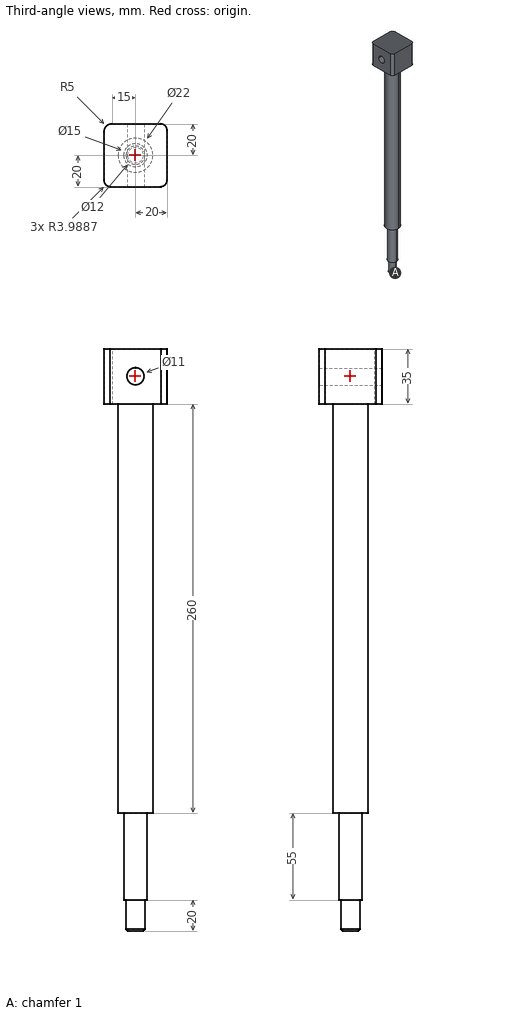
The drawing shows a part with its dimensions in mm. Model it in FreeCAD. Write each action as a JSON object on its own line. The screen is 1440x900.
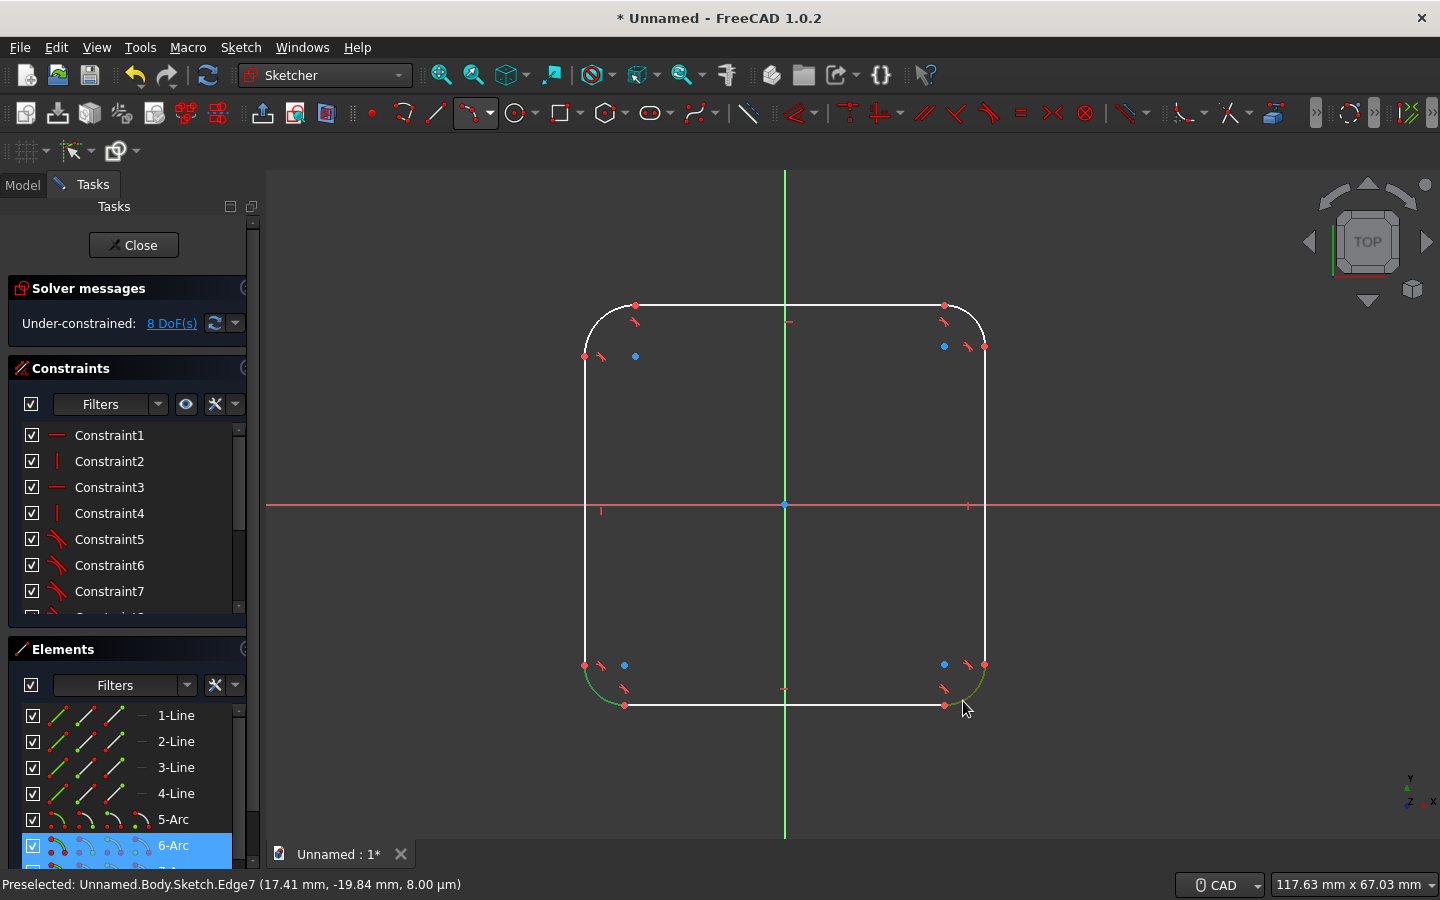
{"action": "left_click", "coordinate": [981, 328]}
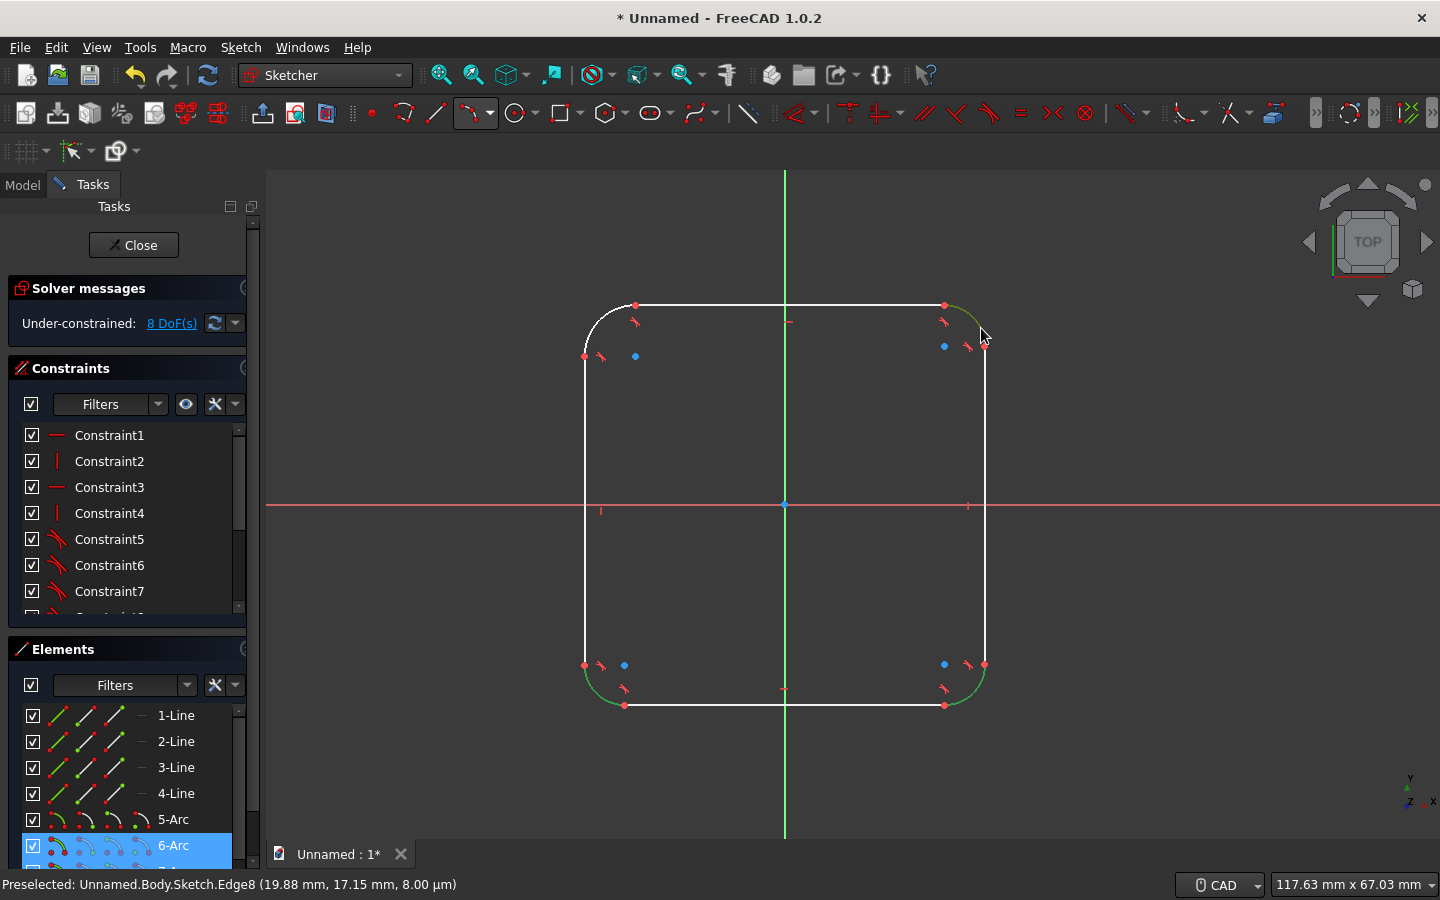
{"action": "left_click", "coordinate": [1022, 114]}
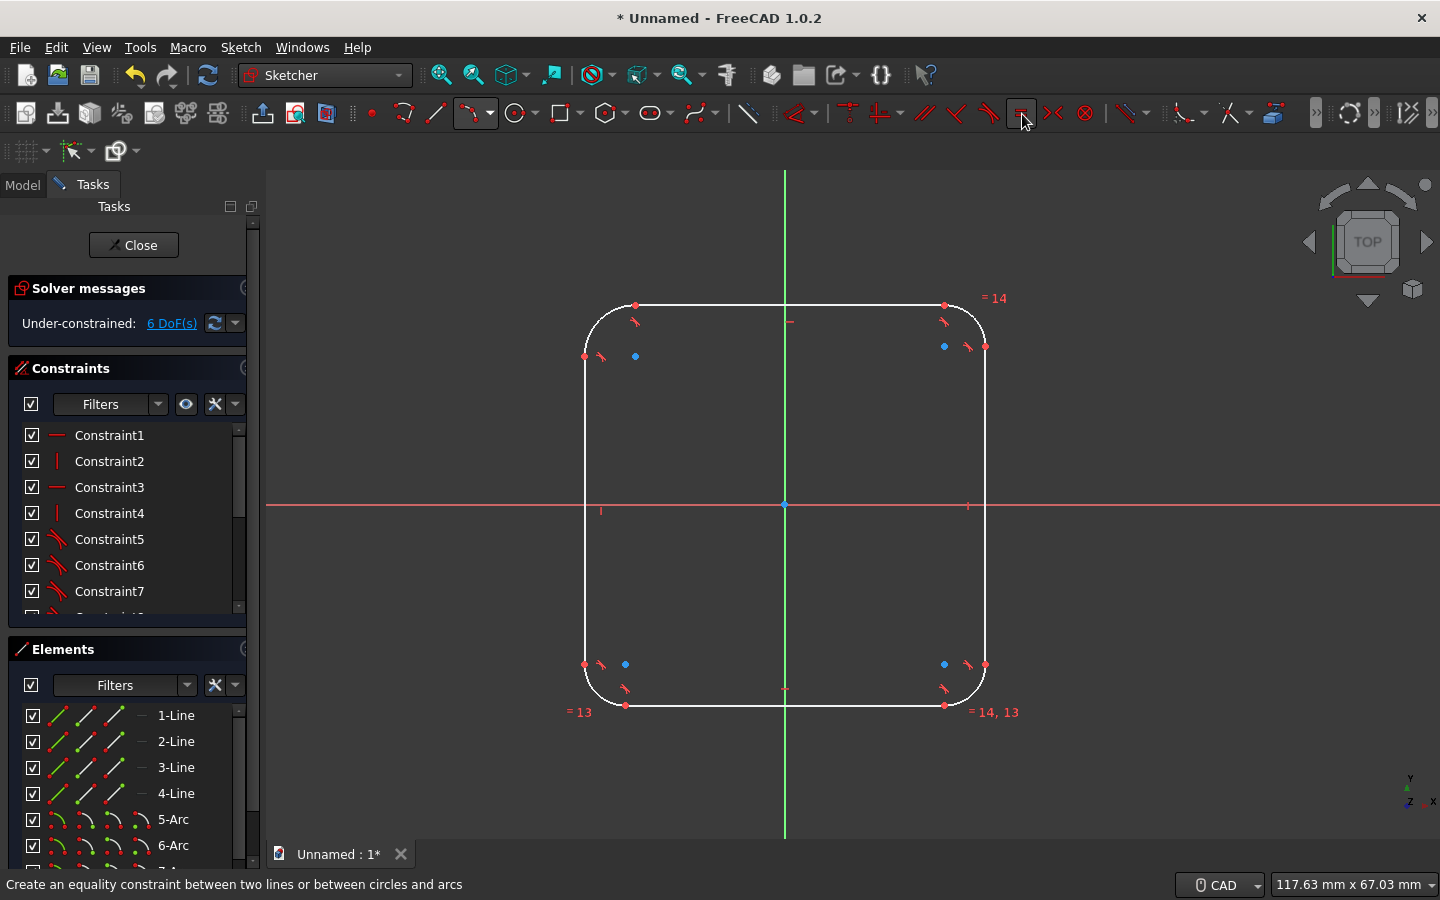
{"action": "left_click", "coordinate": [613, 311]}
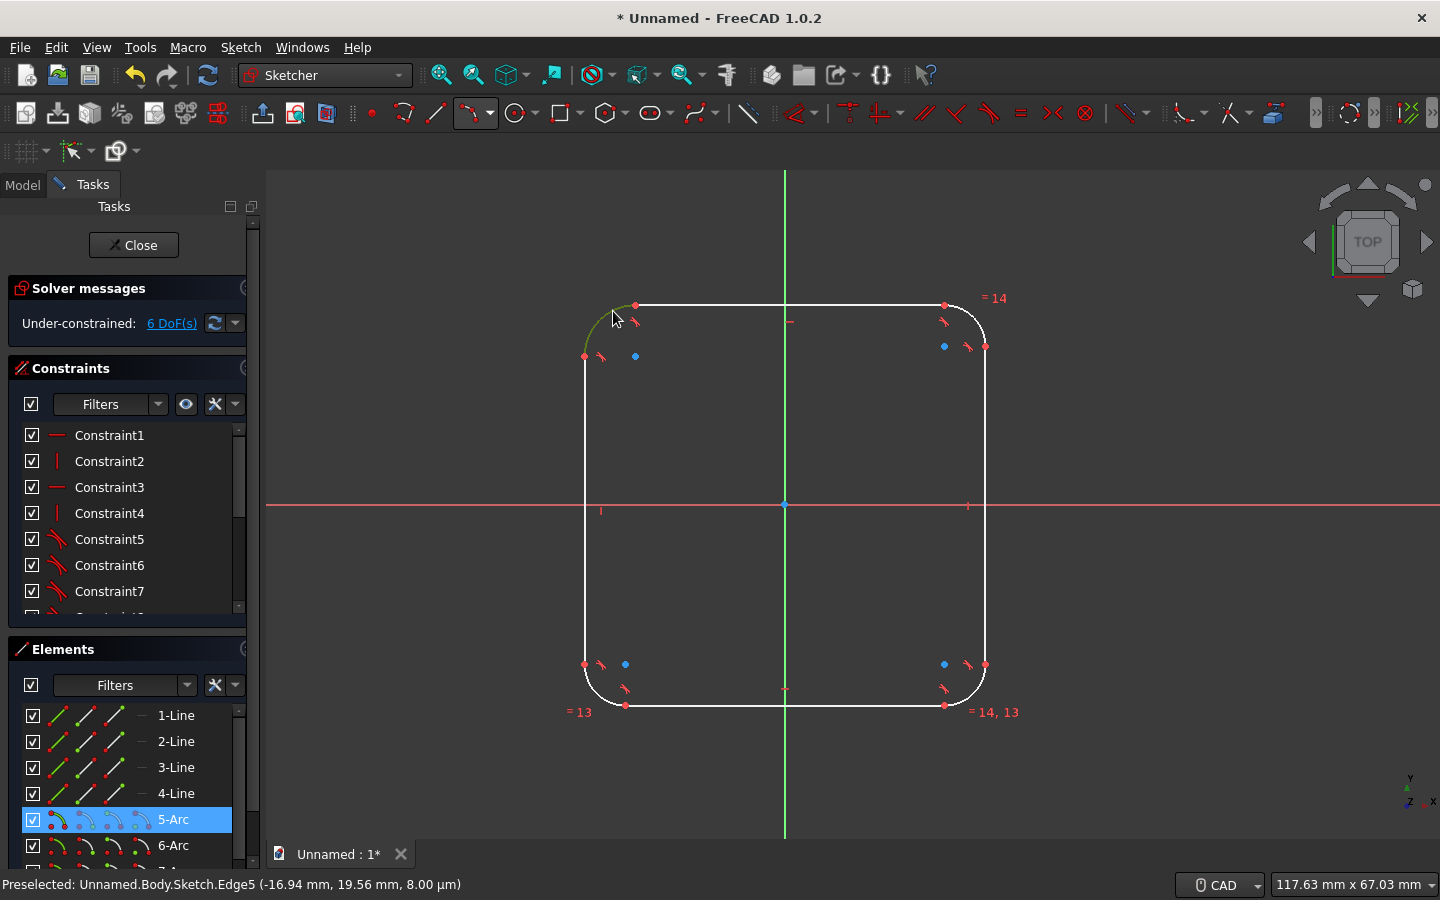
{"action": "key", "text": "k r"}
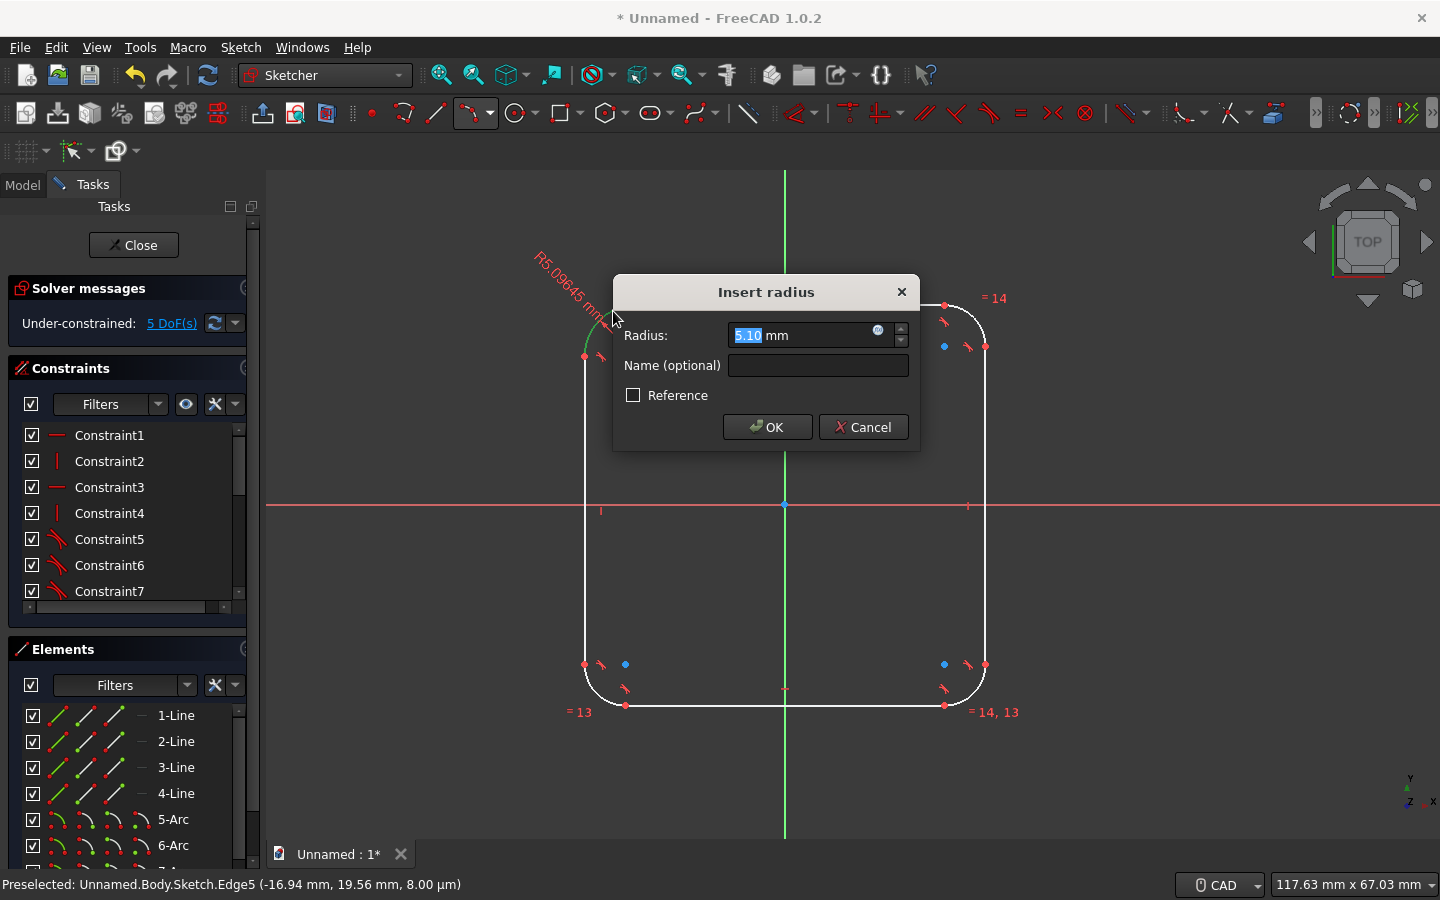
{"action": "type", "text": "5"}
{"action": "key", "text": "Return"}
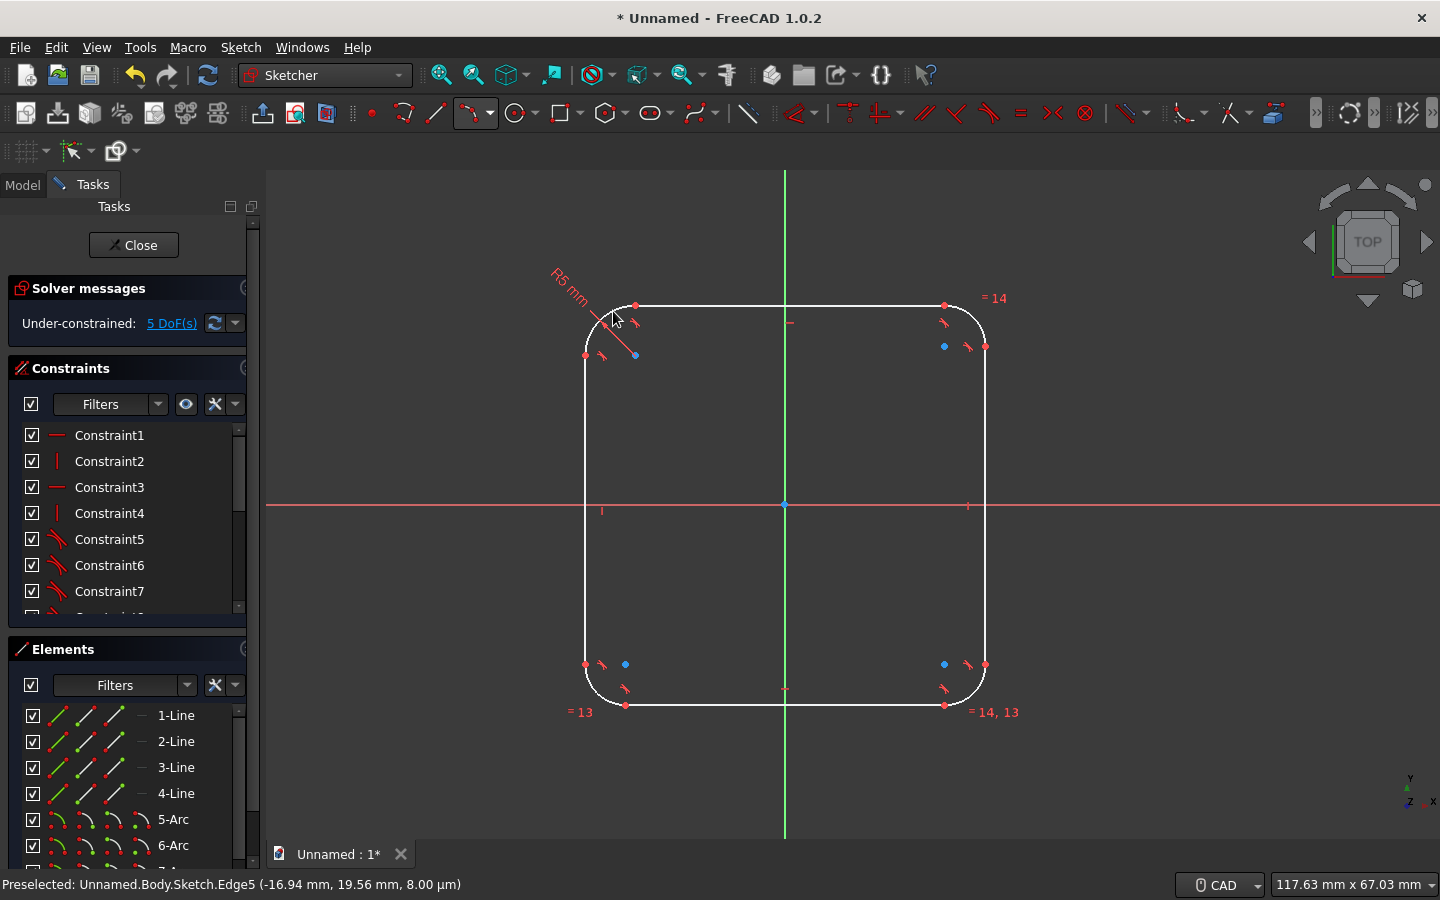
{"action": "left_click", "coordinate": [590, 683]}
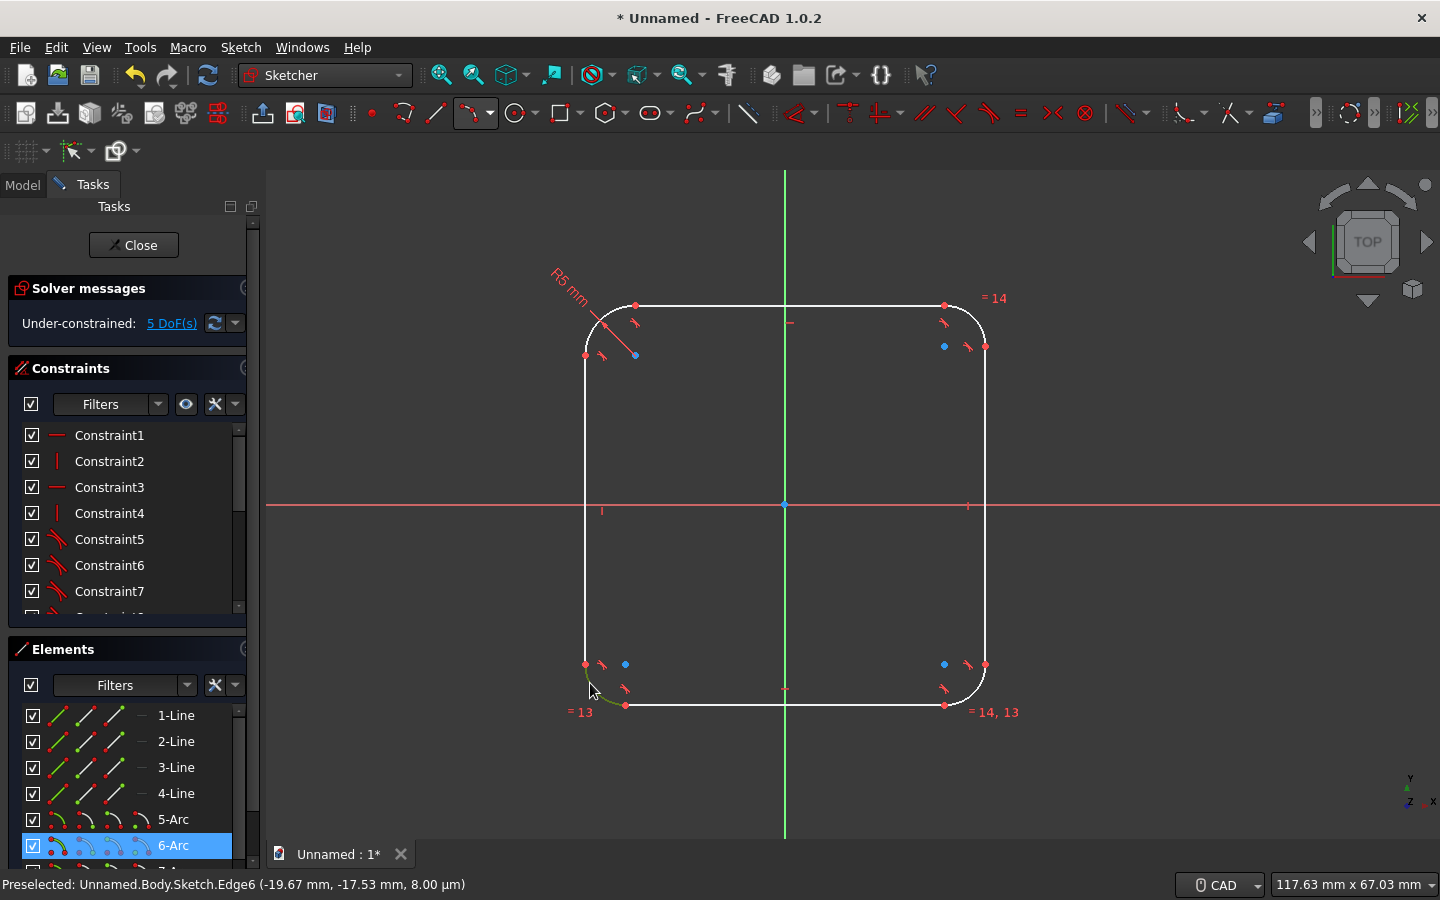
{"action": "key", "text": "k r"}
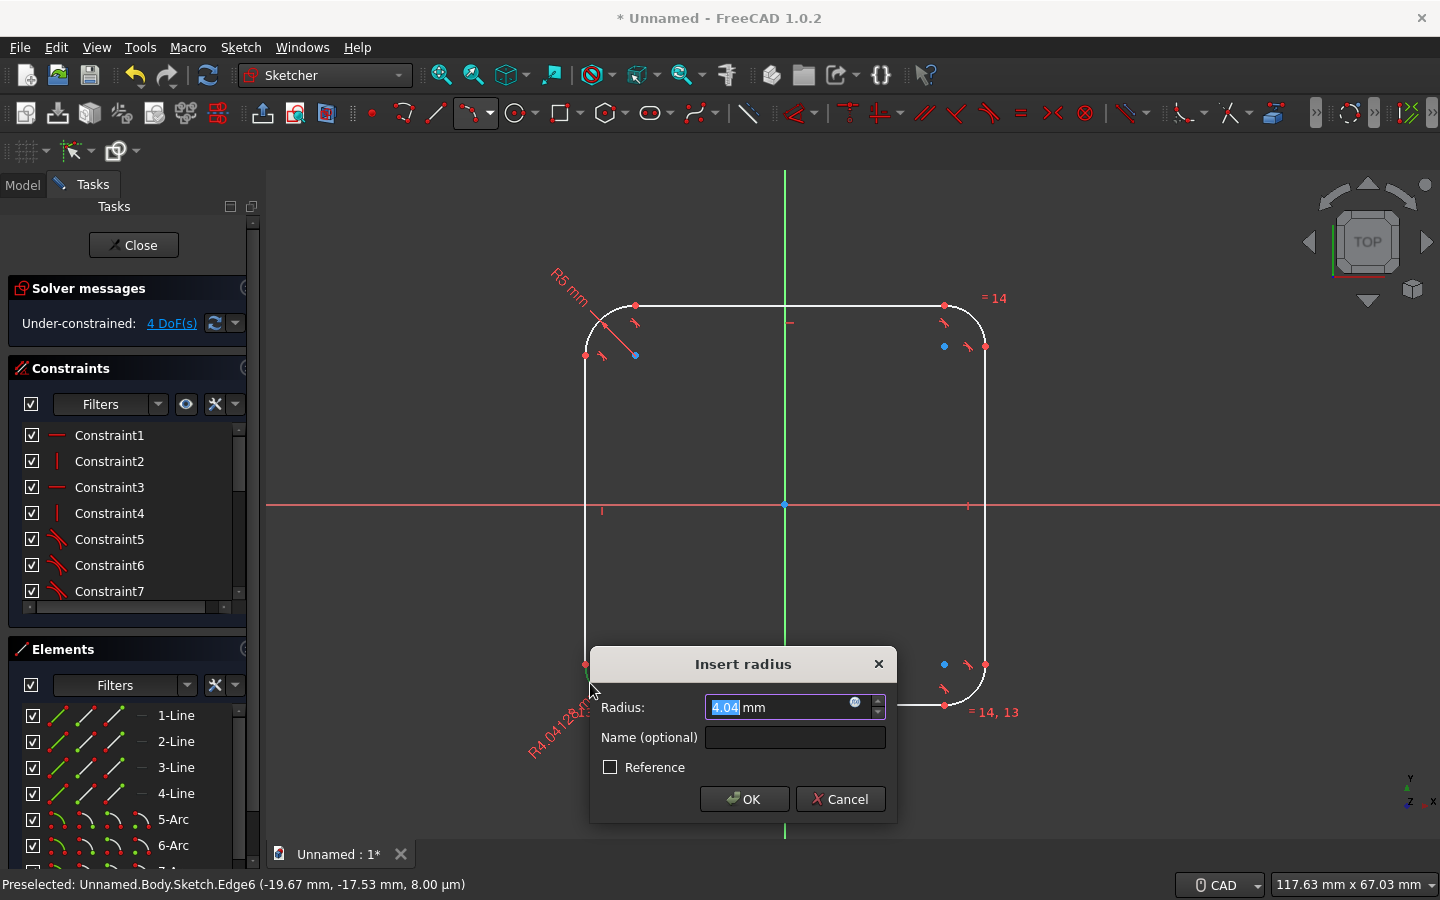
{"action": "type", "text": "3.9887"}
{"action": "key", "text": "Return"}